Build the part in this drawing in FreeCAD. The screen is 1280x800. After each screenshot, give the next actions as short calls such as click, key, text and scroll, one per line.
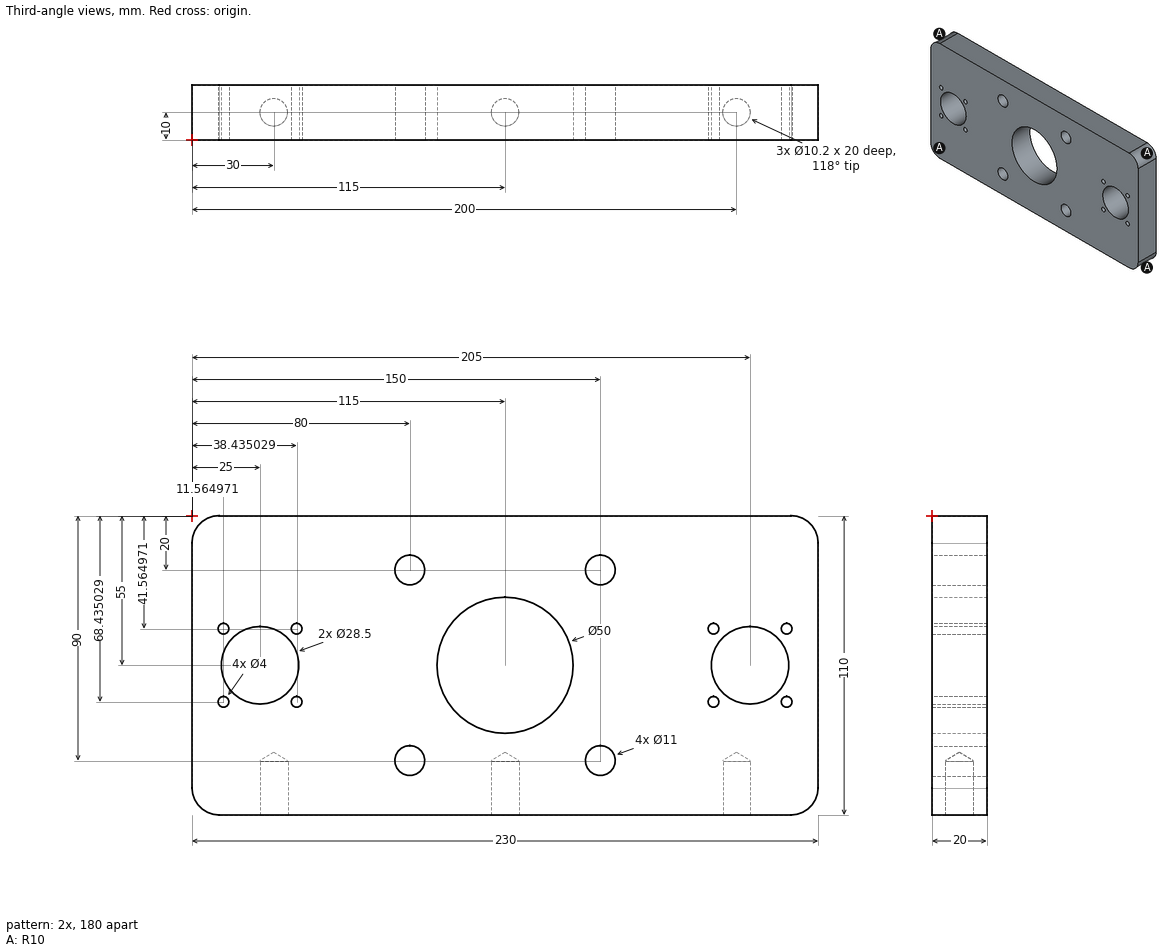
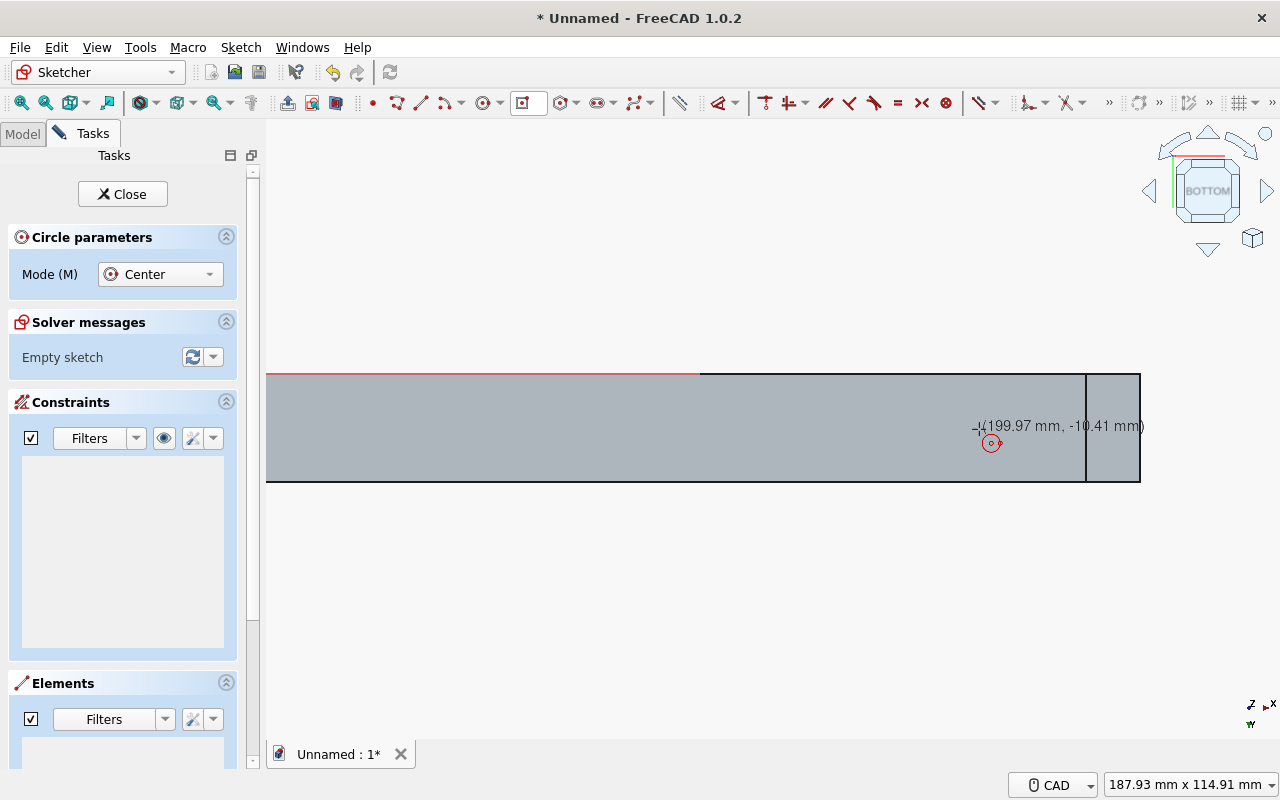
click(978, 428)
move(998, 409)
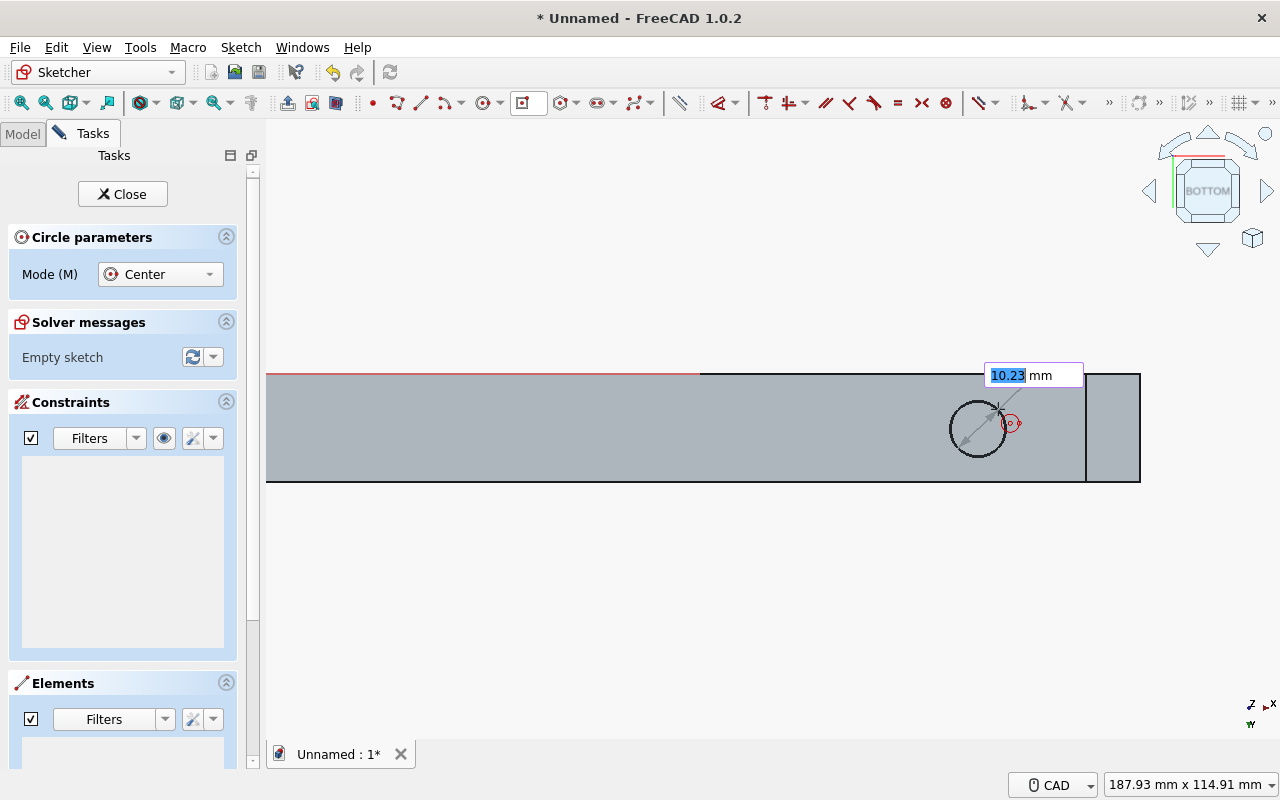
text(10.2)
key(Return)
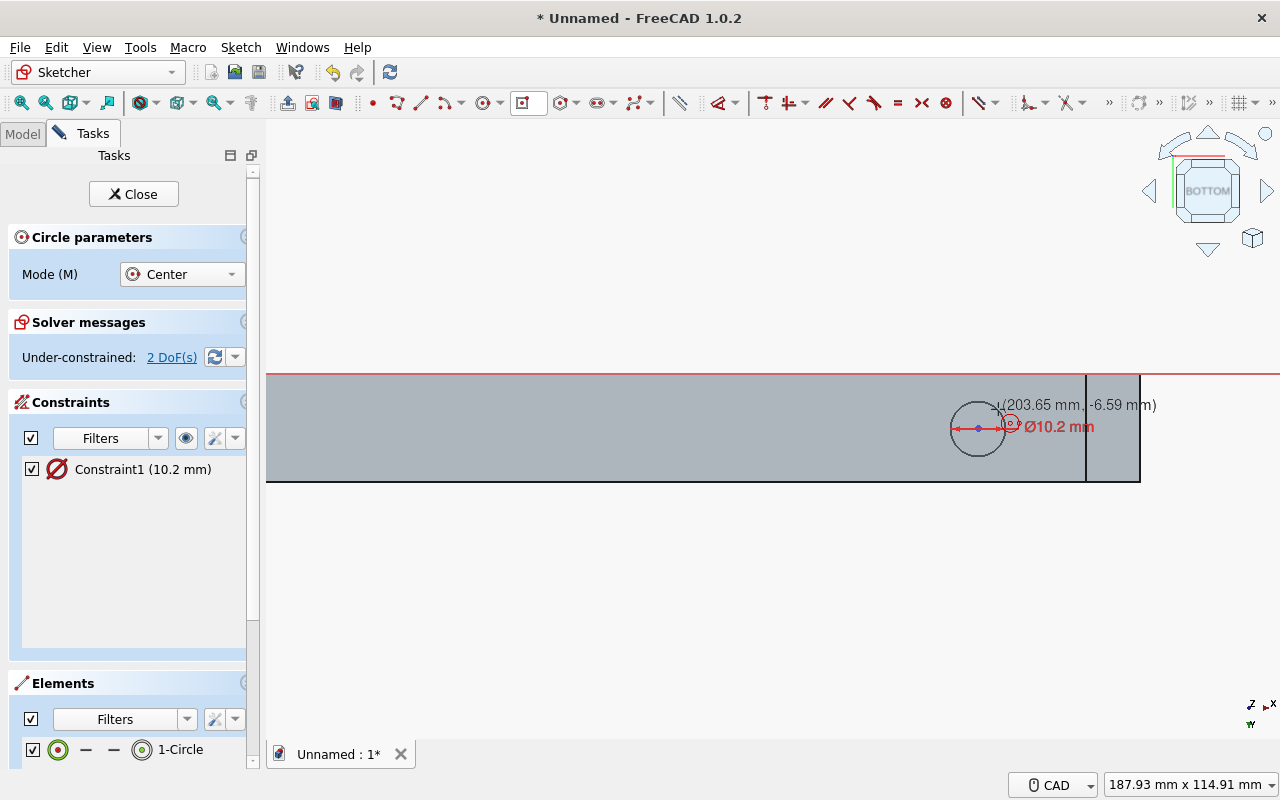
click(520, 428)
move(539, 409)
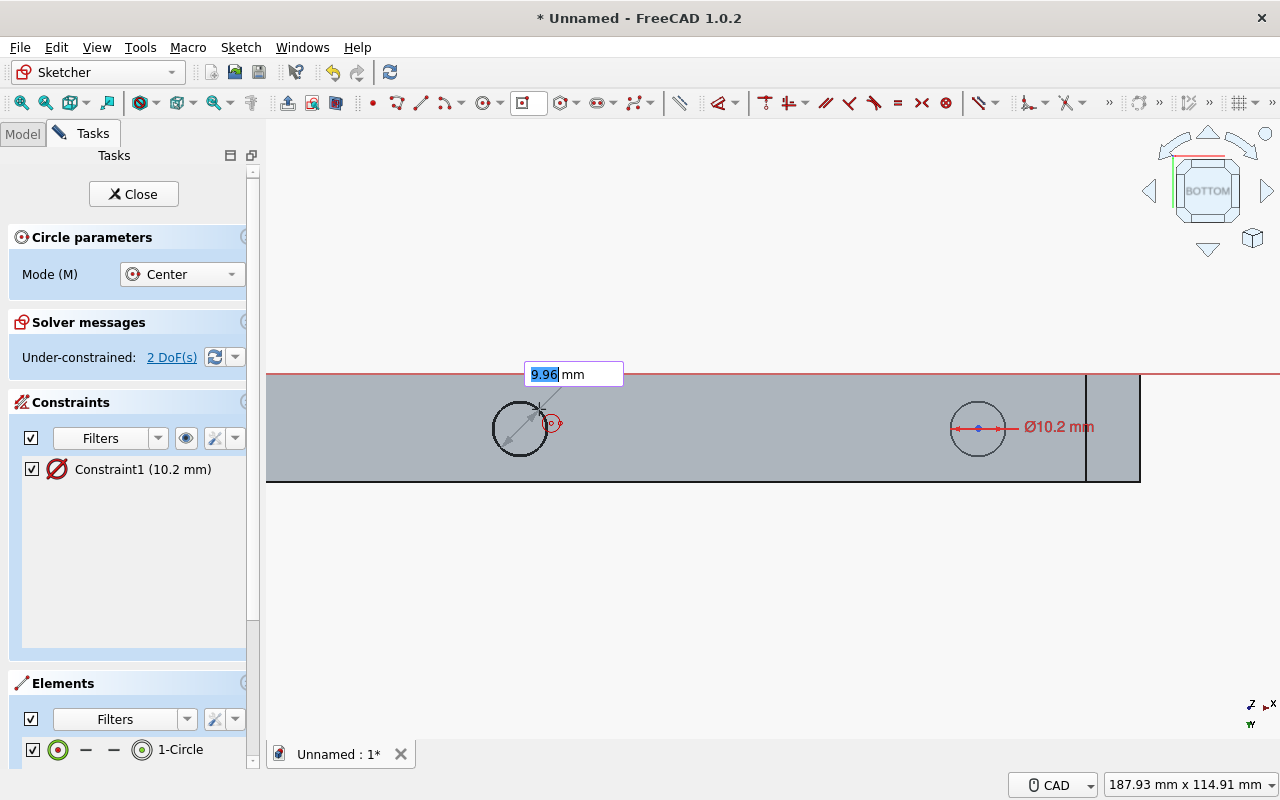
text(10.2)
key(Return)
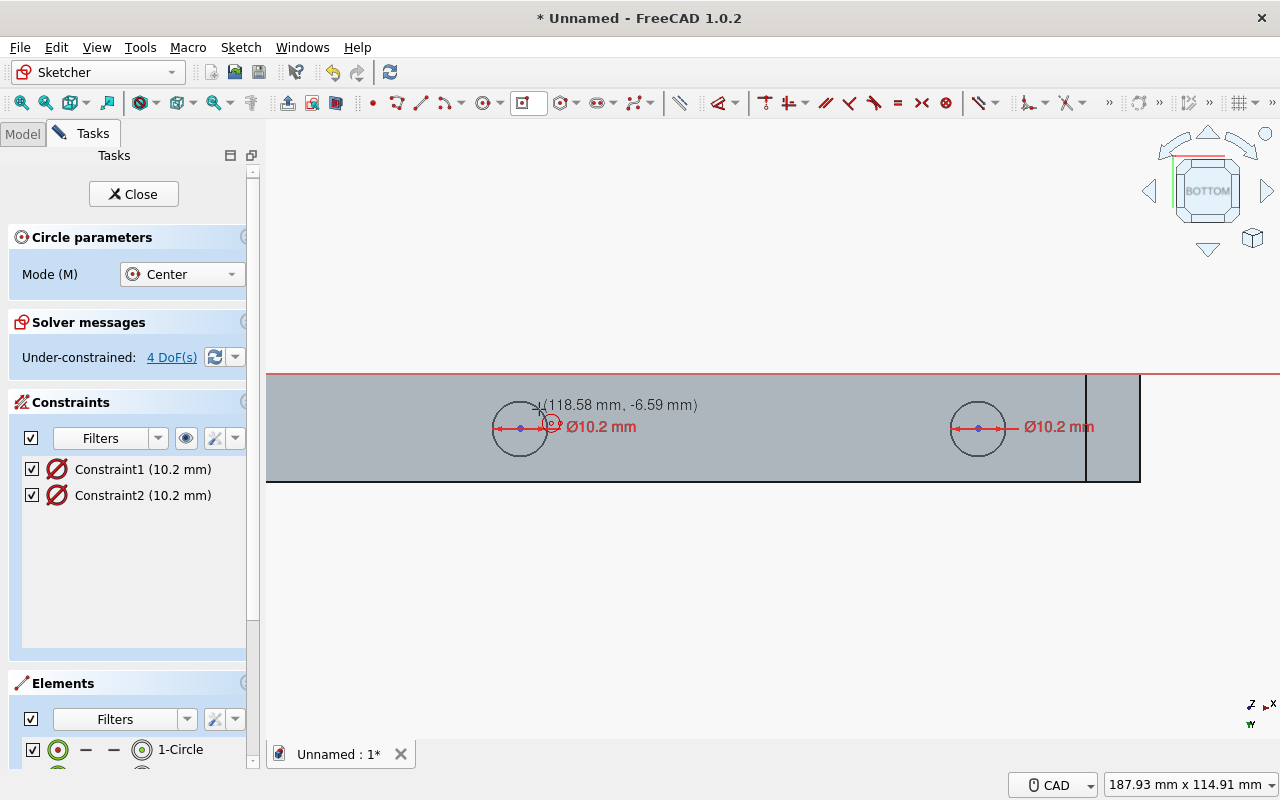
scroll(1011, 446, down, 3)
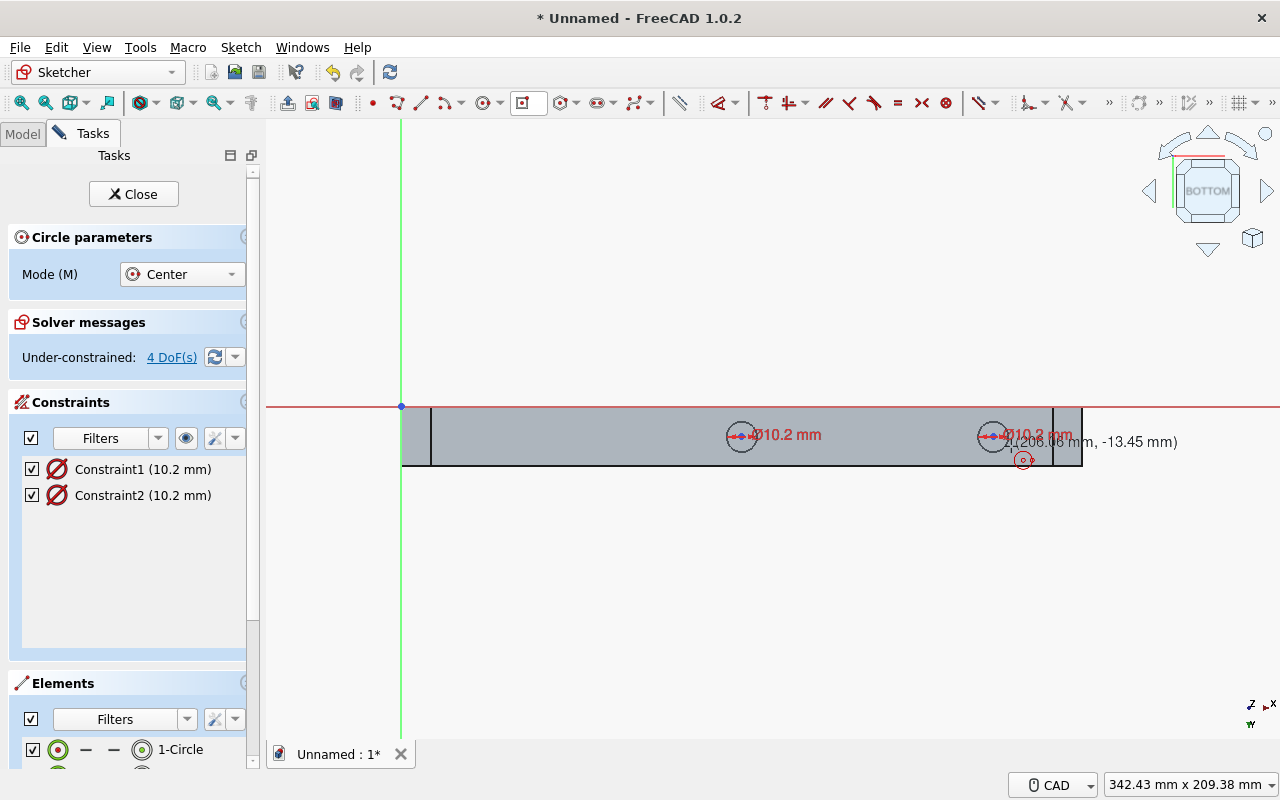
scroll(490, 437, up, 3)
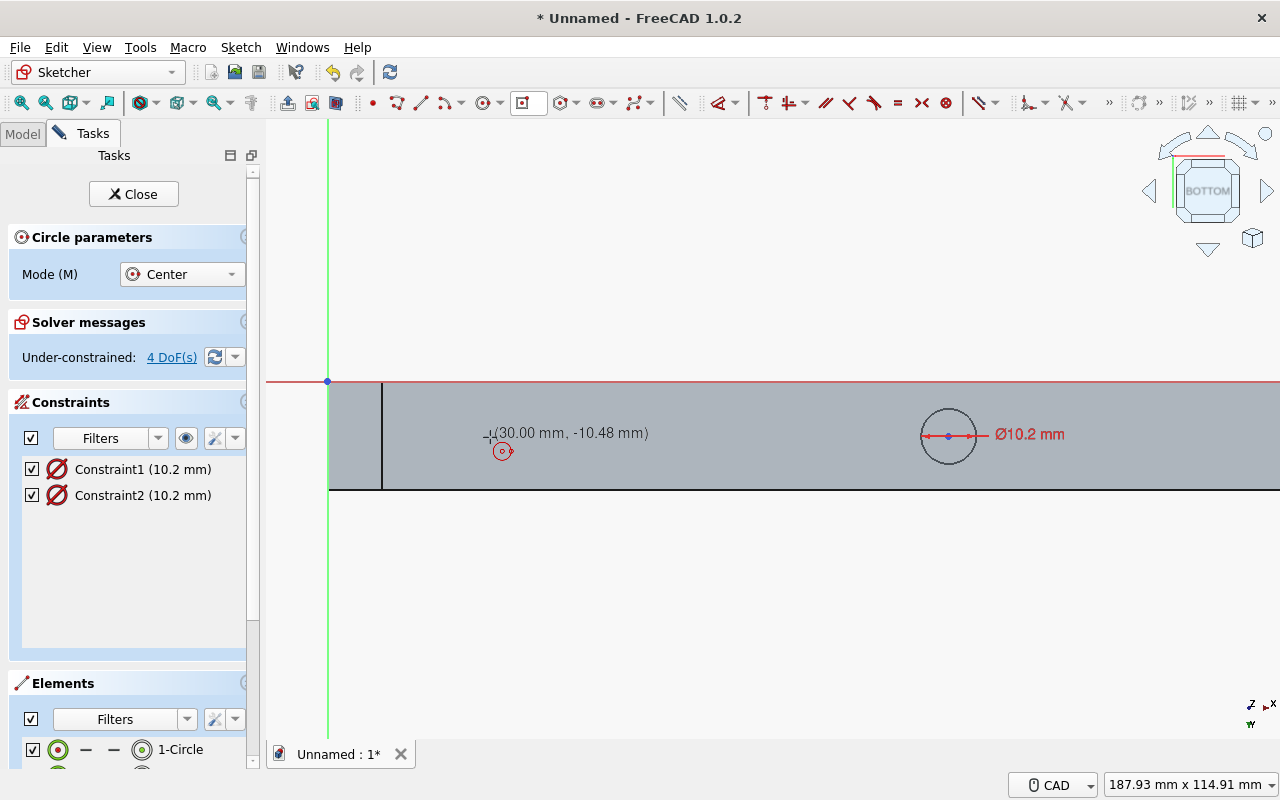
click(490, 436)
move(509, 416)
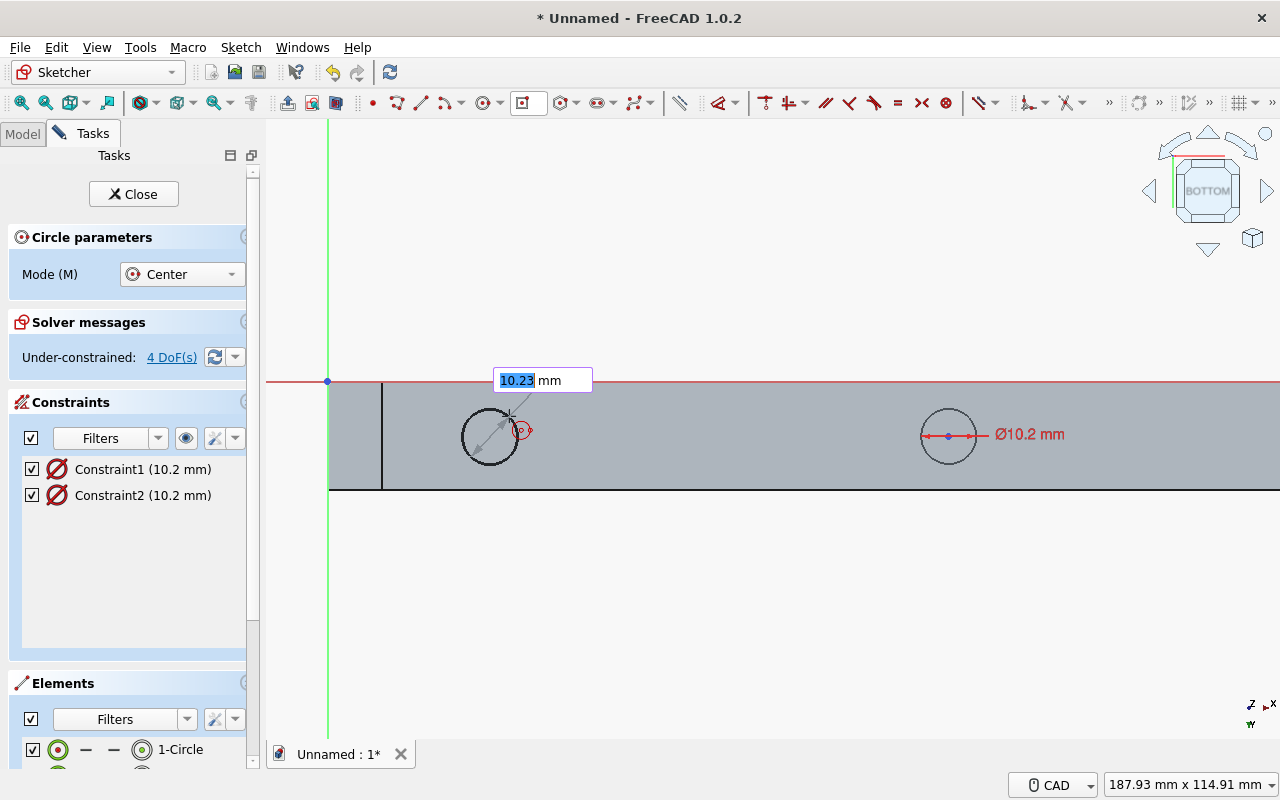
text(10.2)
key(Return)
key(Escape)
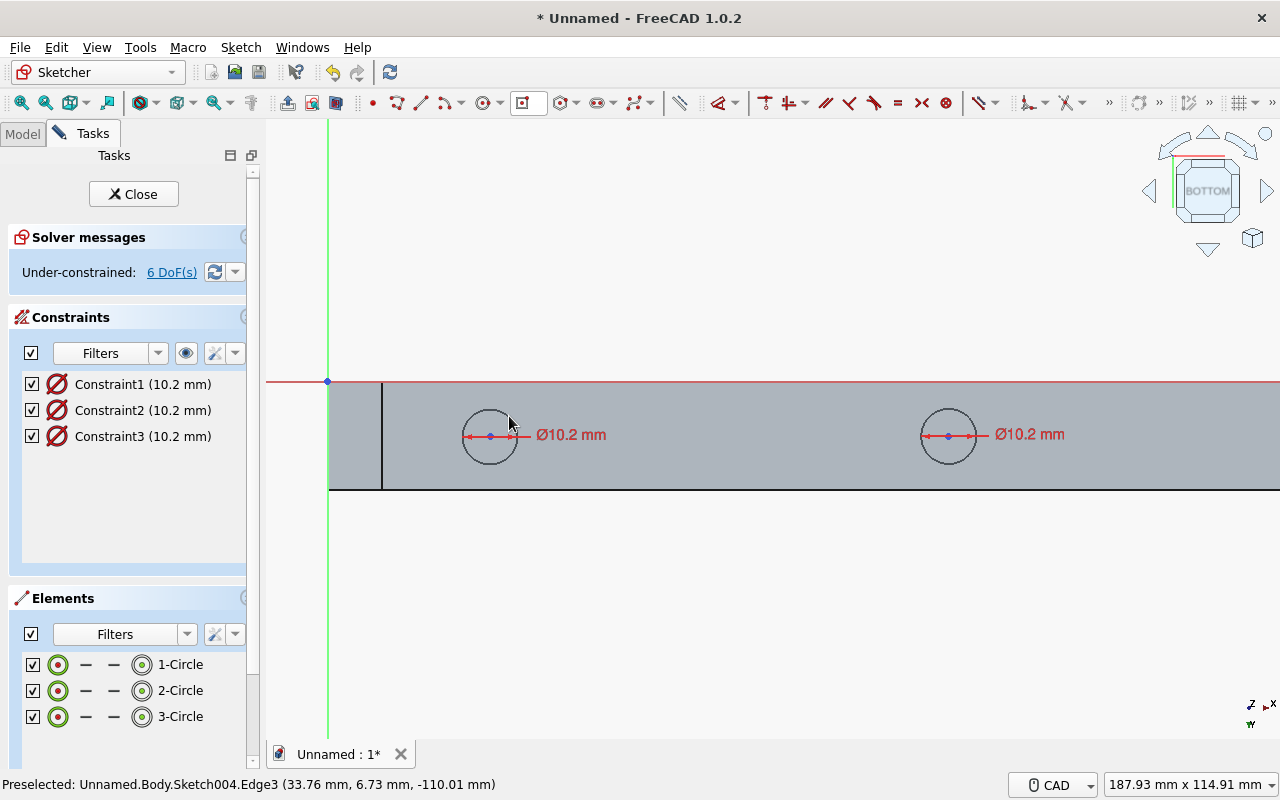
key(d)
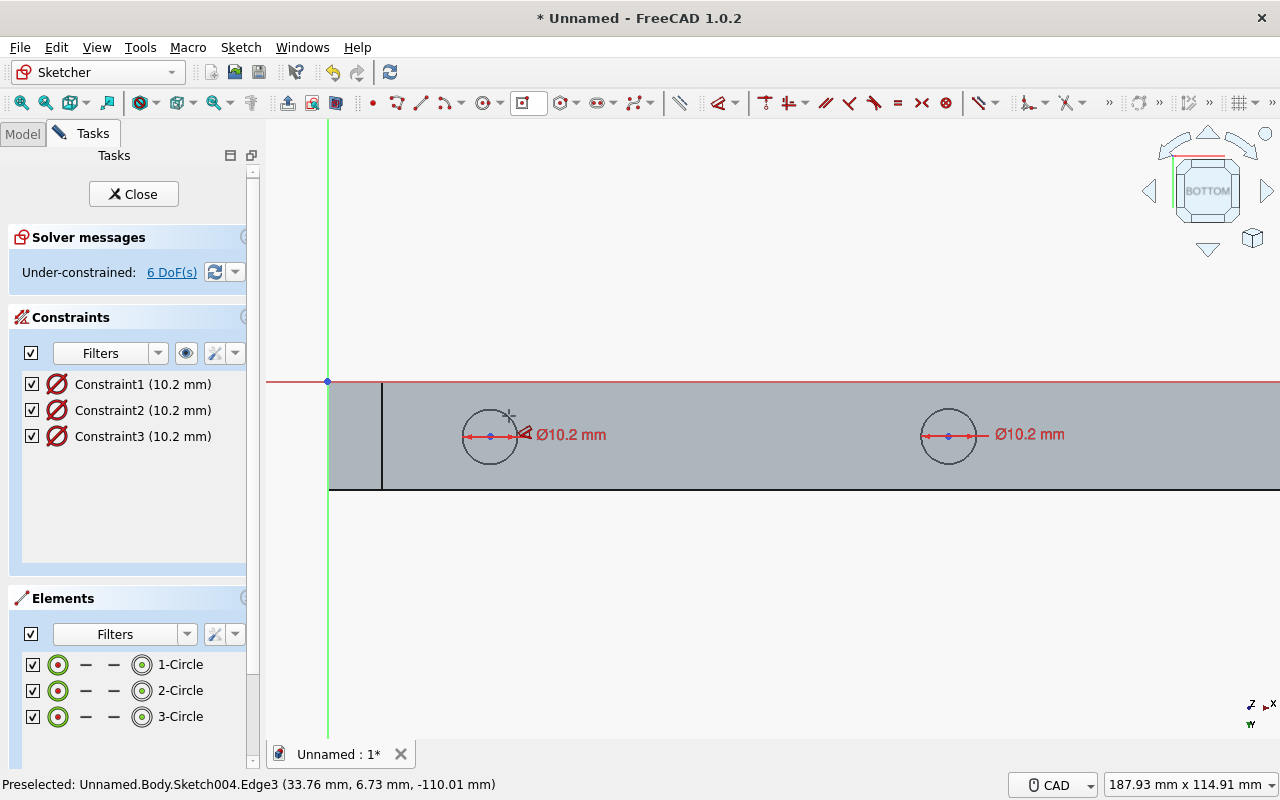
scroll(490, 437, down, 3)